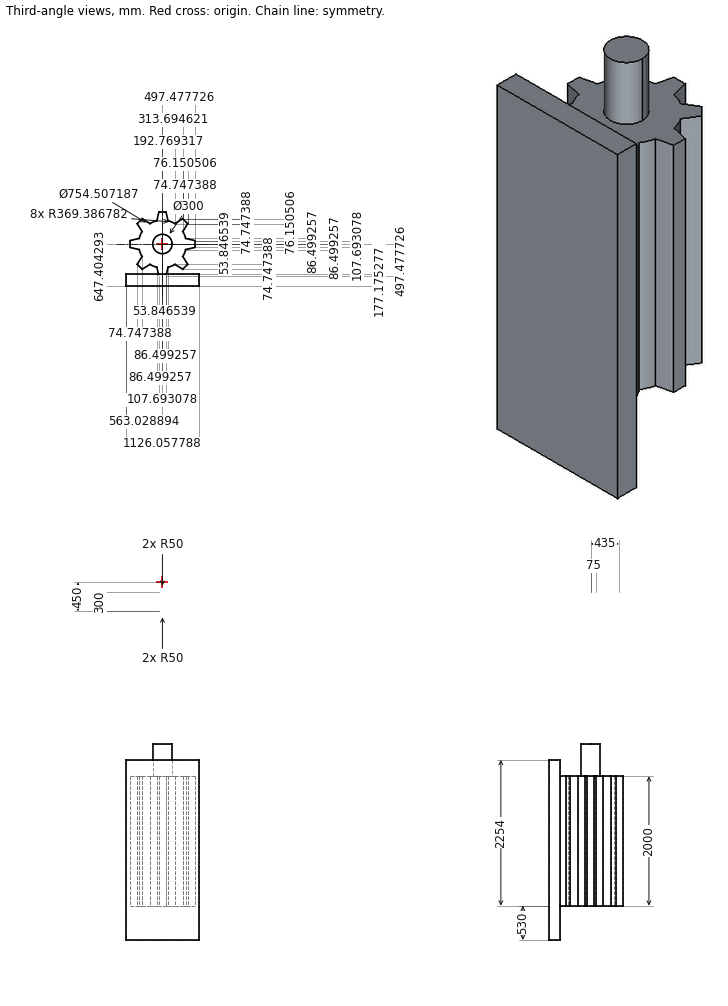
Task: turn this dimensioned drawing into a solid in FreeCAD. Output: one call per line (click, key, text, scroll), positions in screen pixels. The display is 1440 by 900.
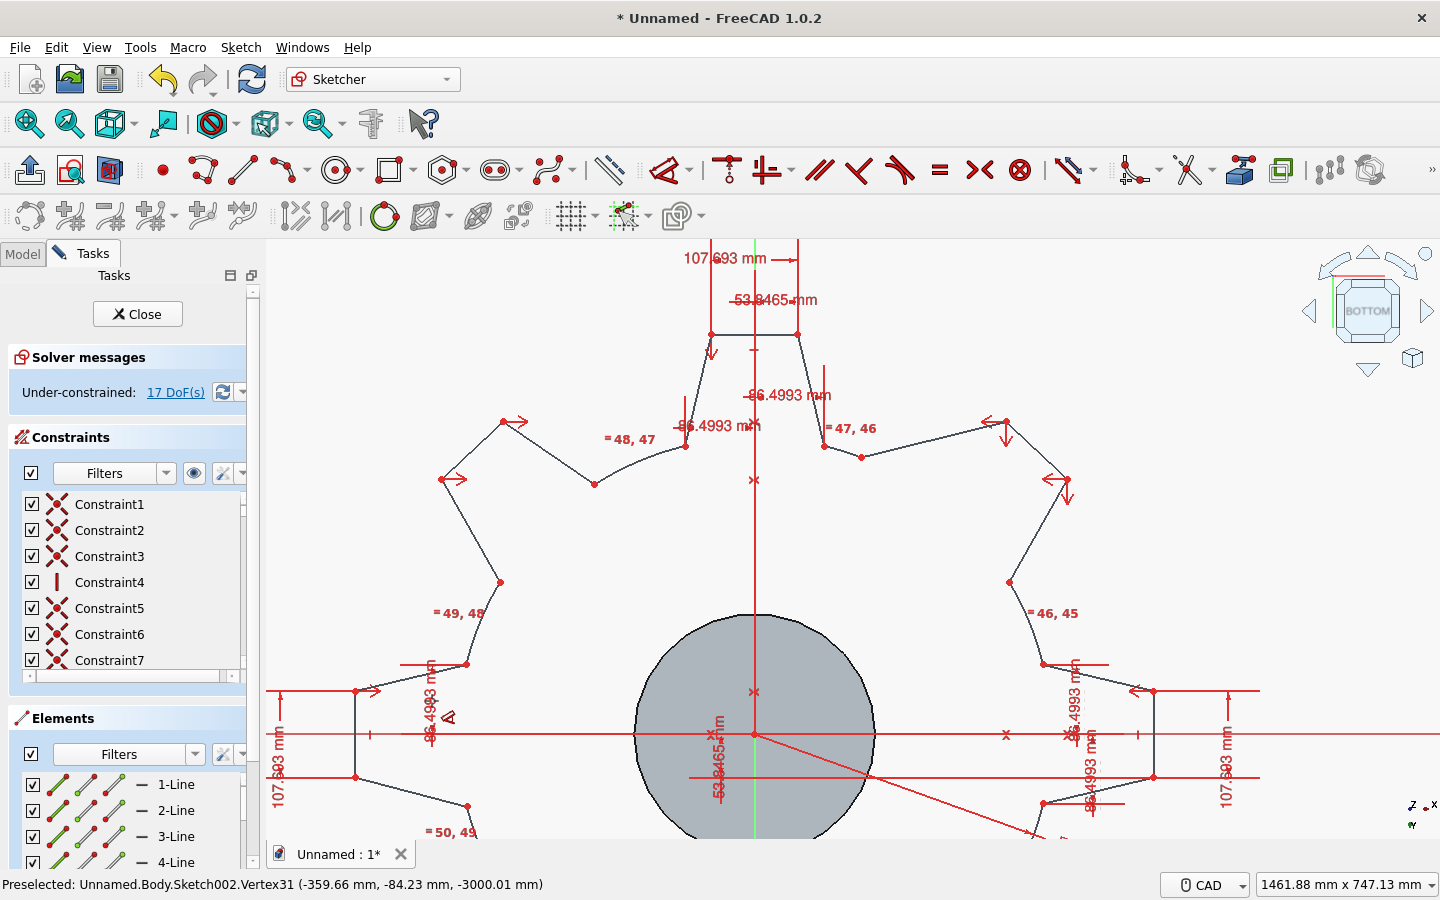
click(467, 807)
click(433, 771)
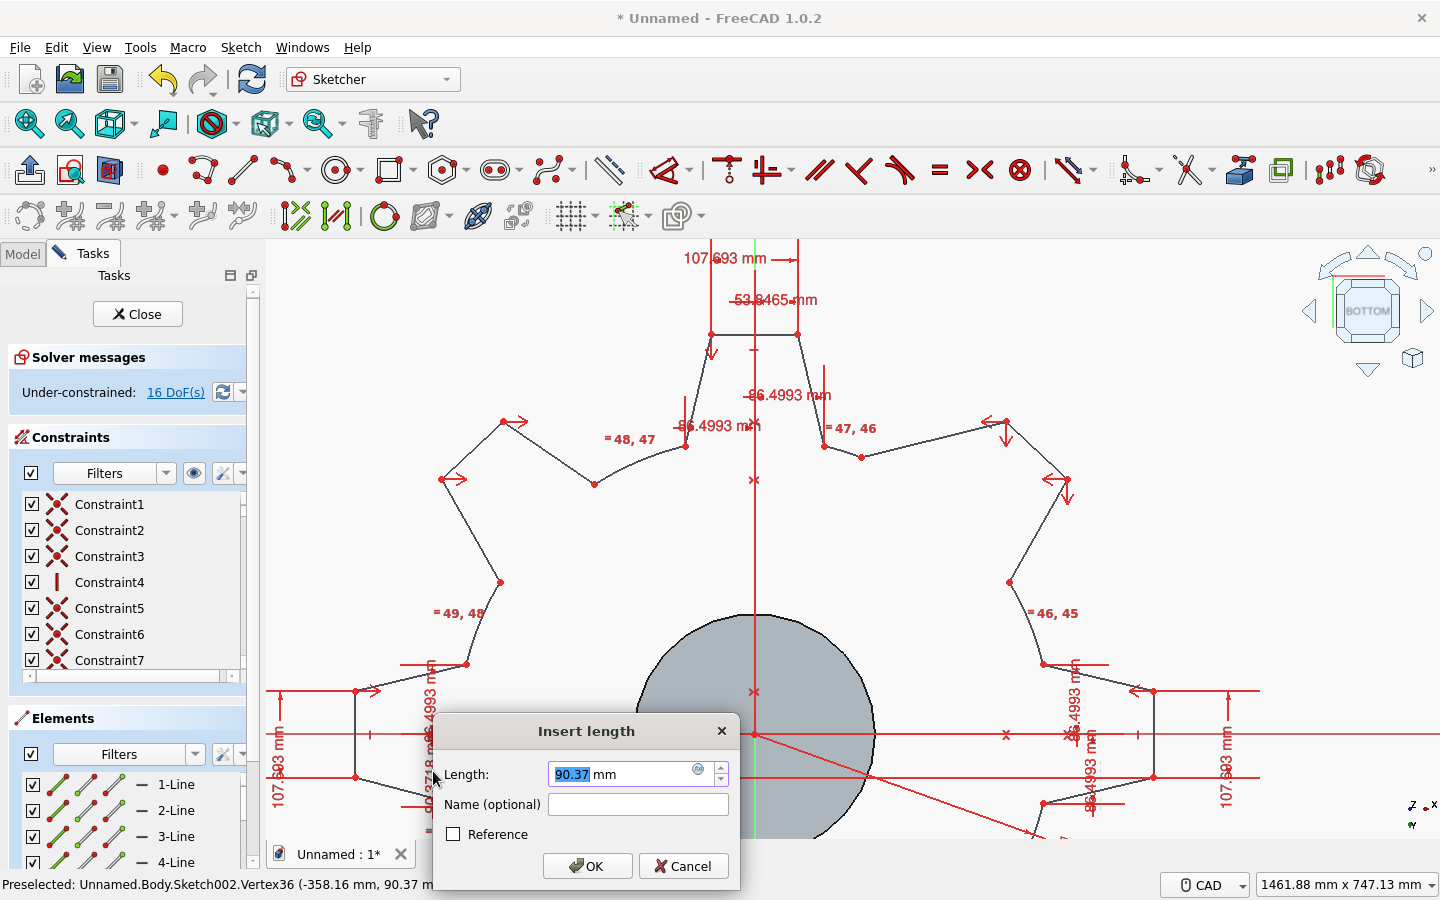
text(86.499257)
key(Return)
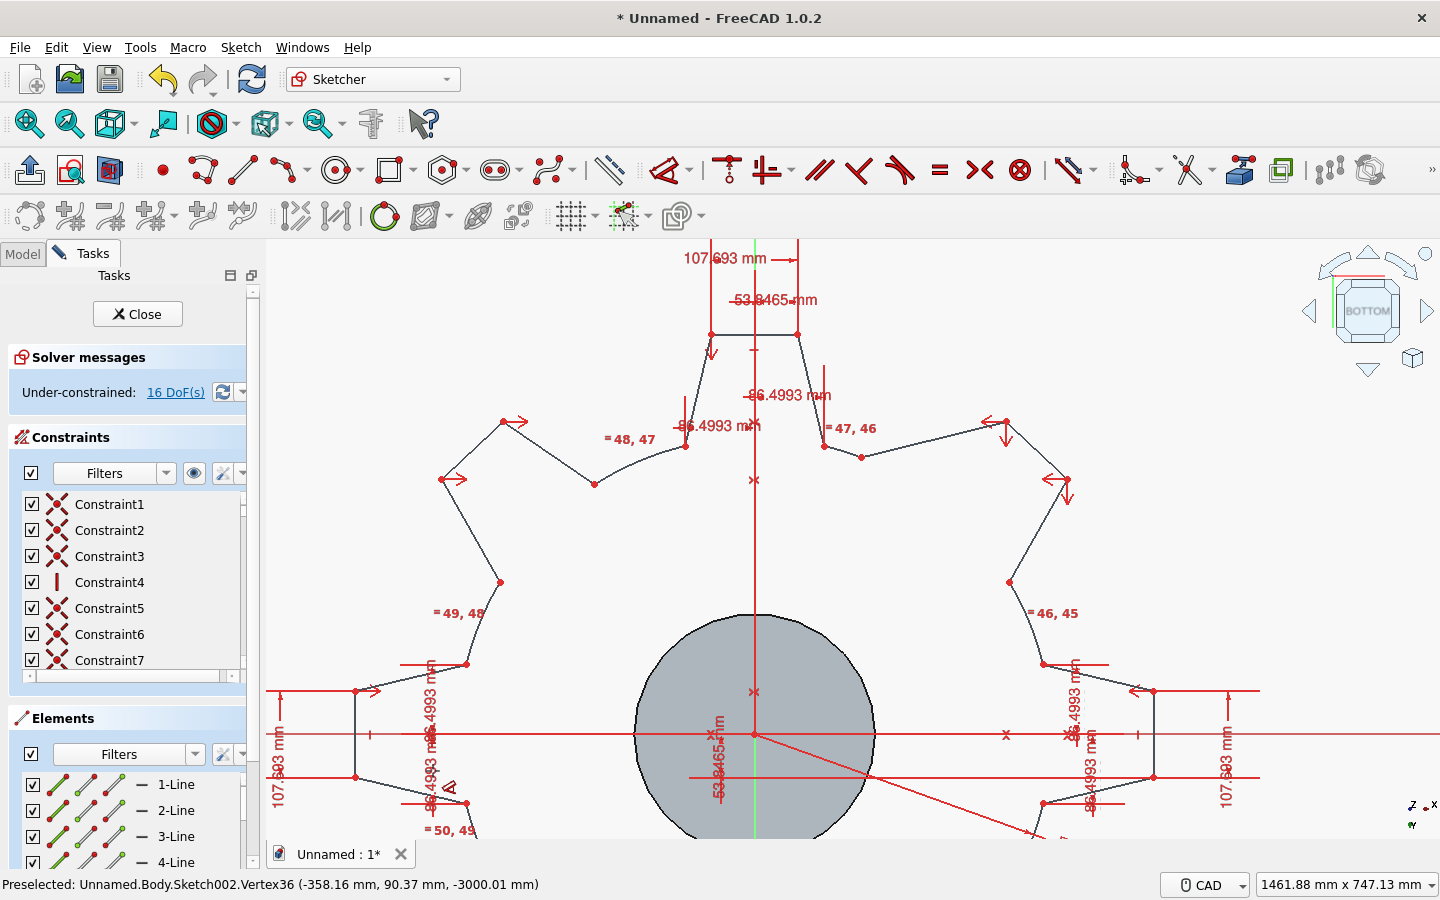
scroll(809, 380, down, 4)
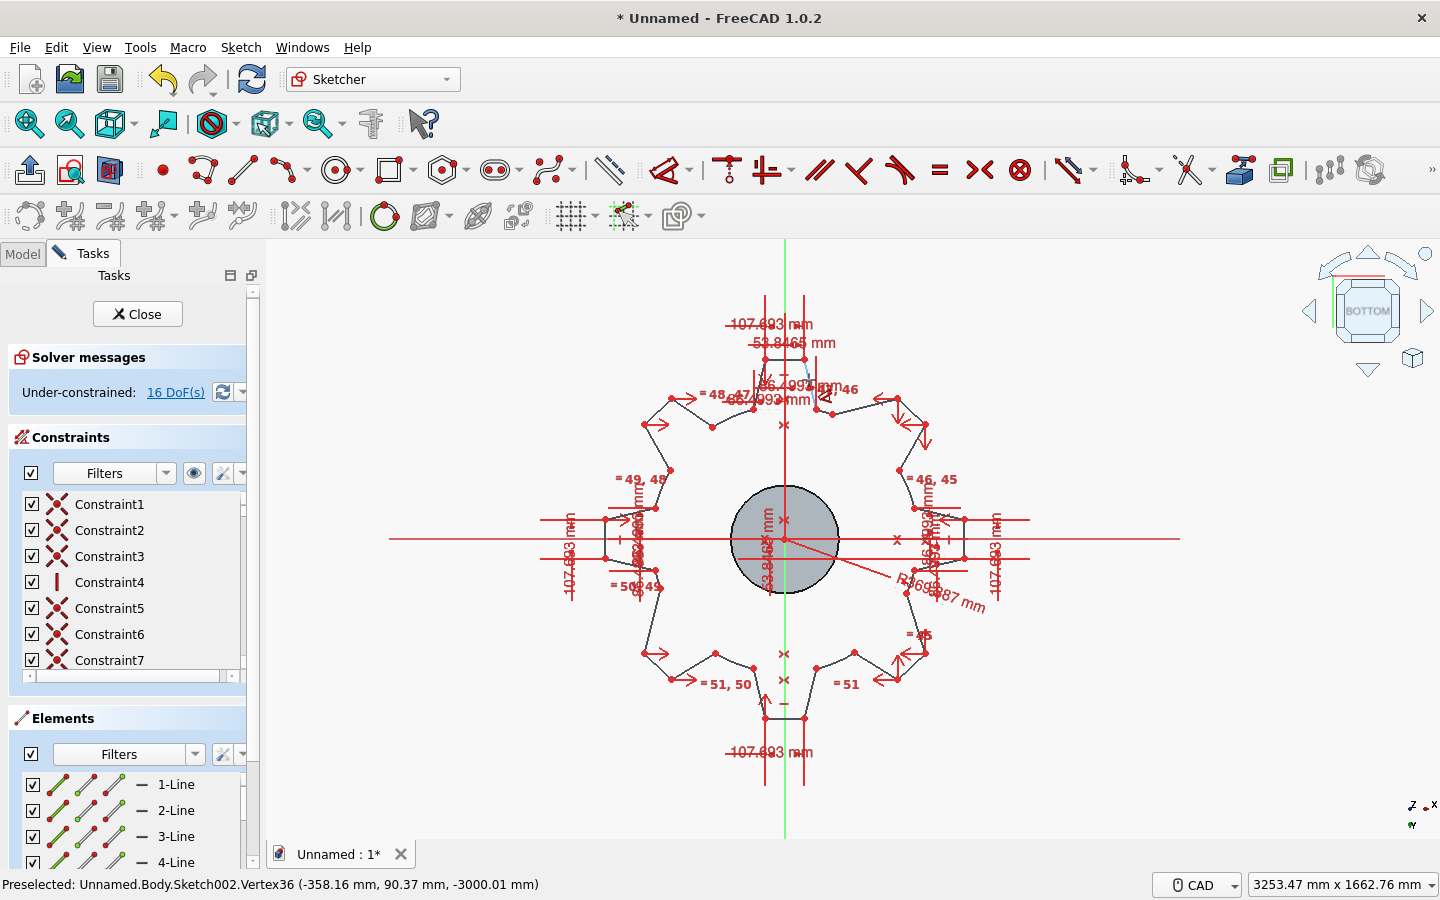
scroll(754, 669, up, 2)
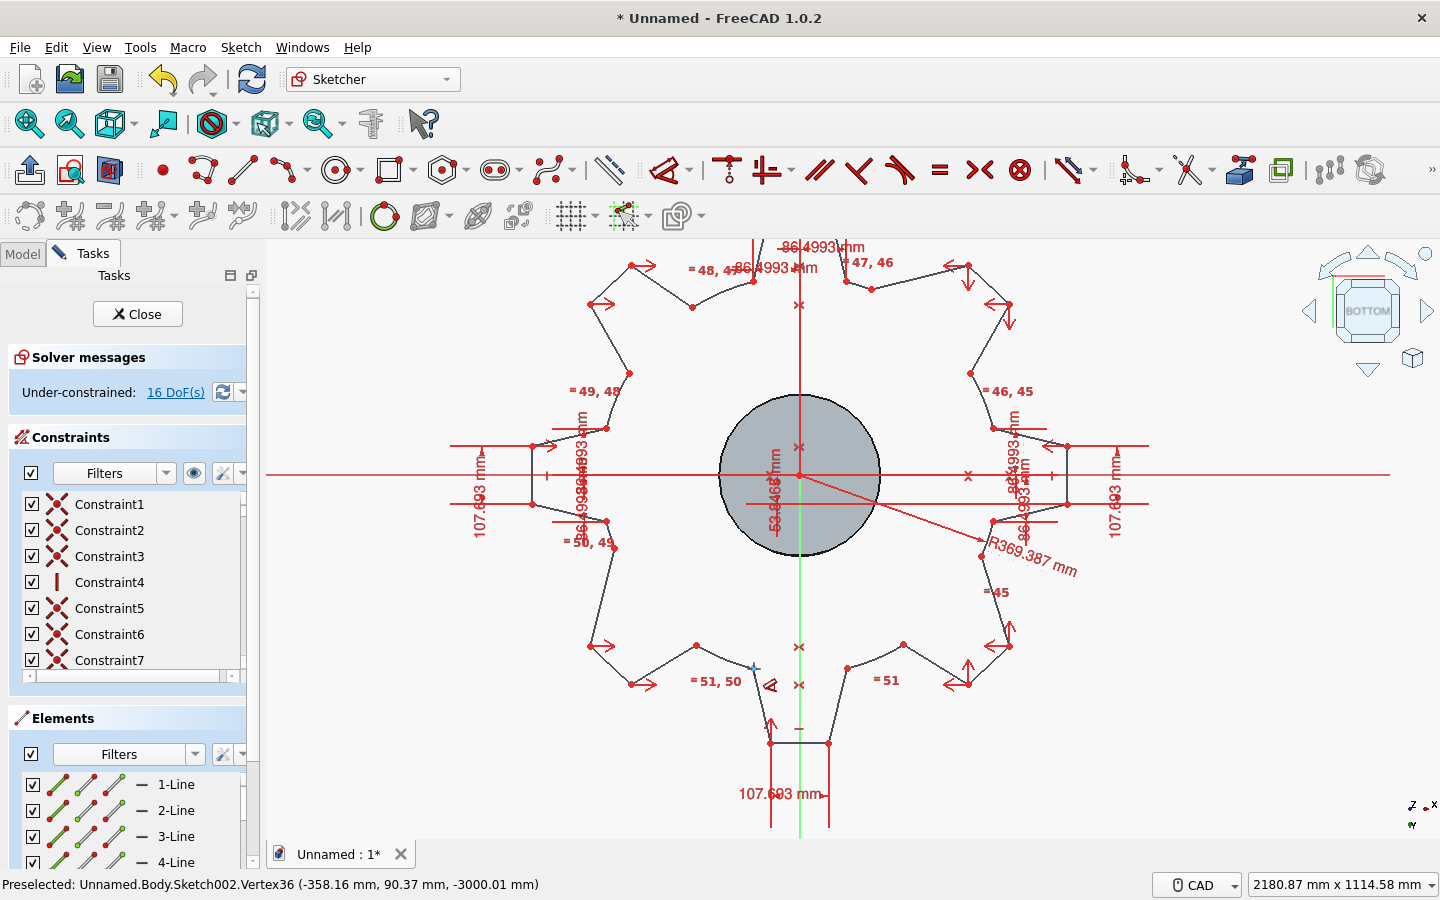
click(753, 669)
click(776, 703)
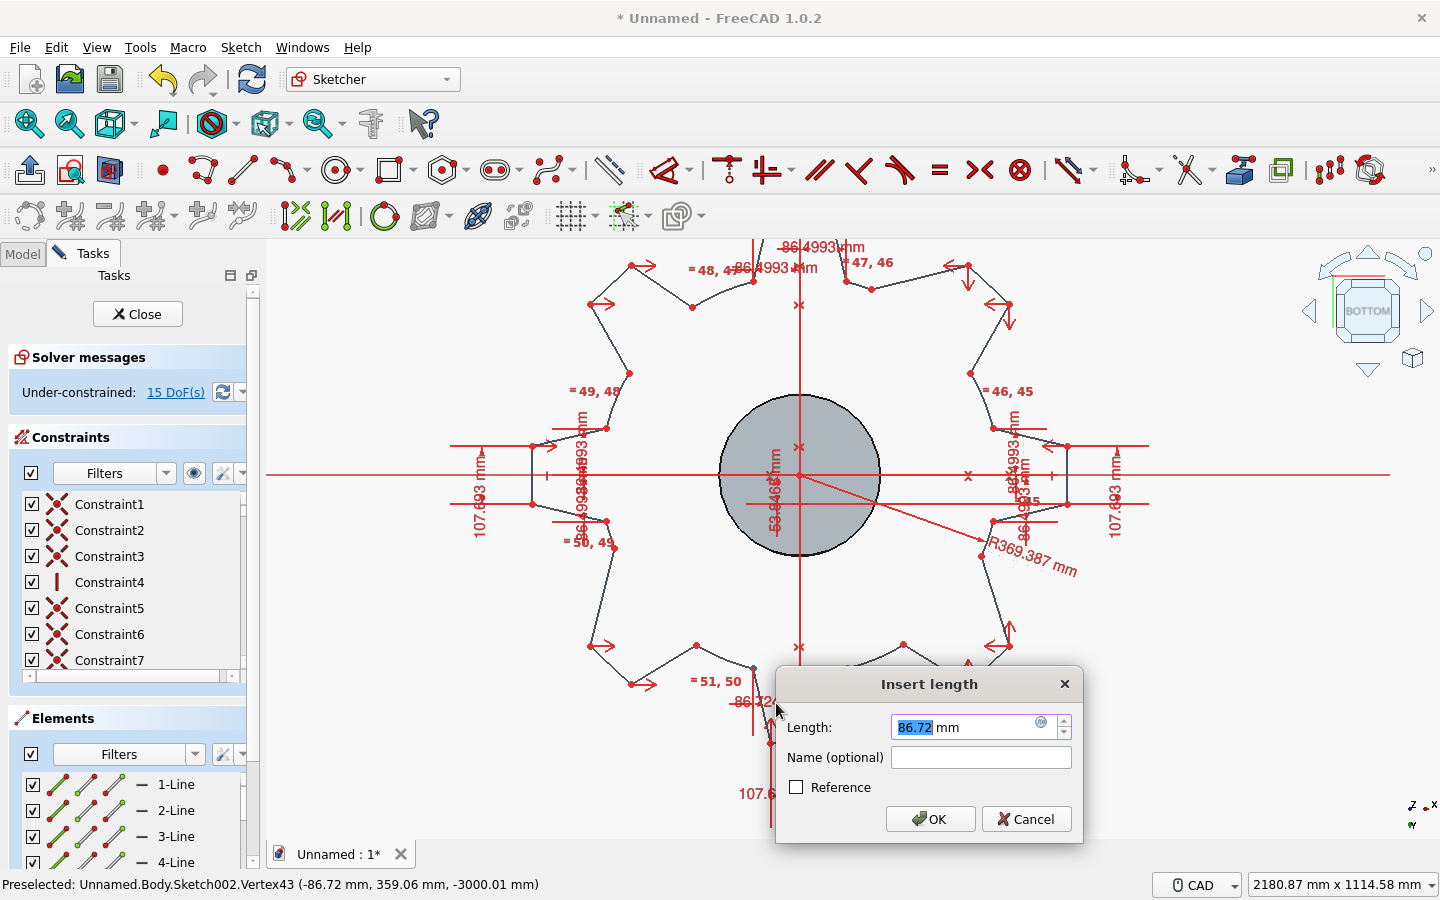
text(86.499257)
key(Return)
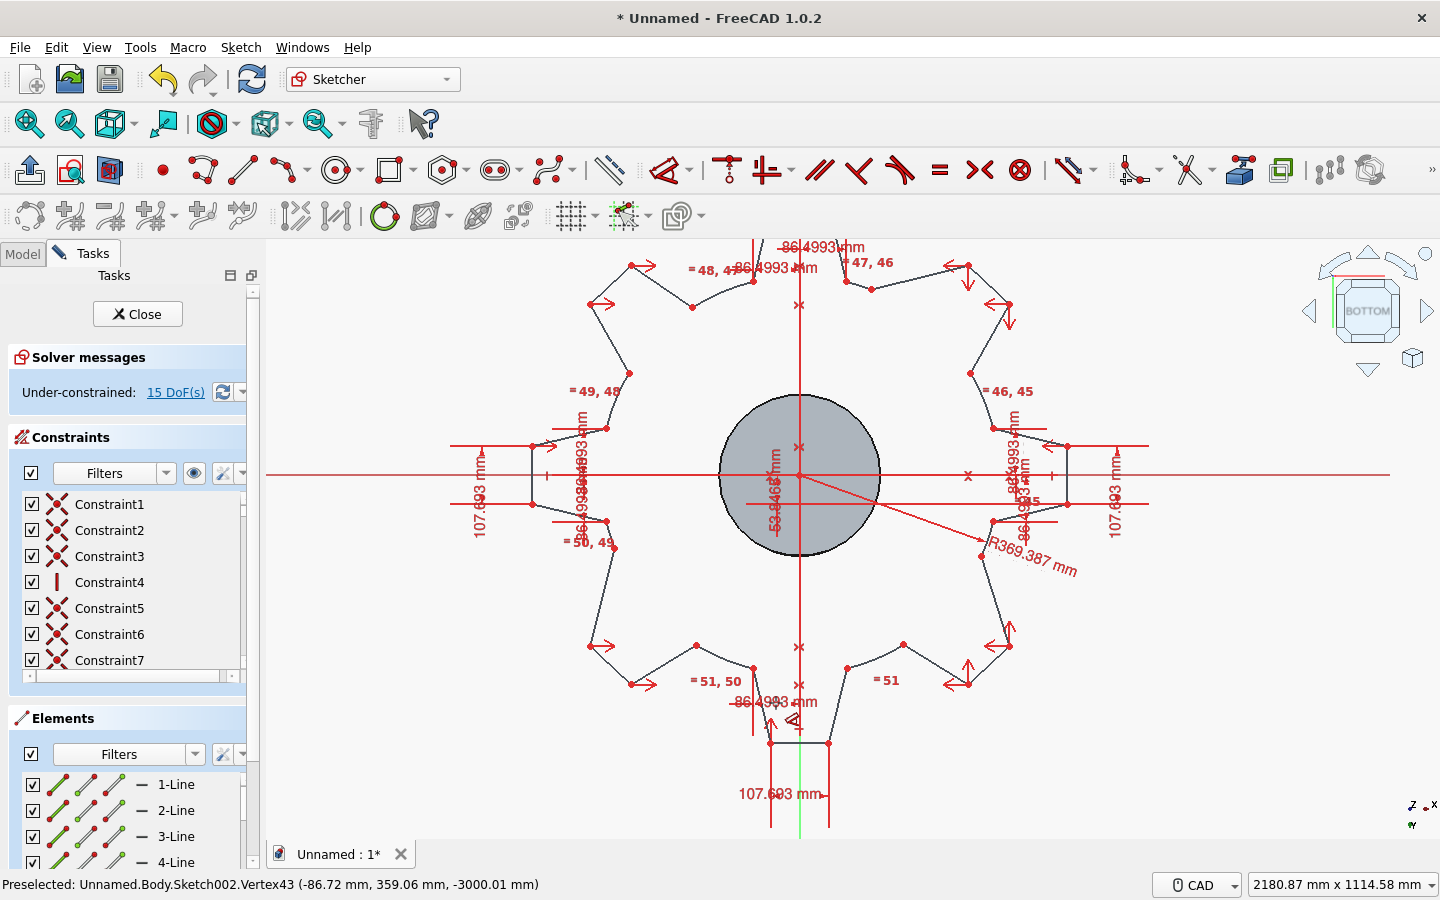
click(847, 668)
click(823, 441)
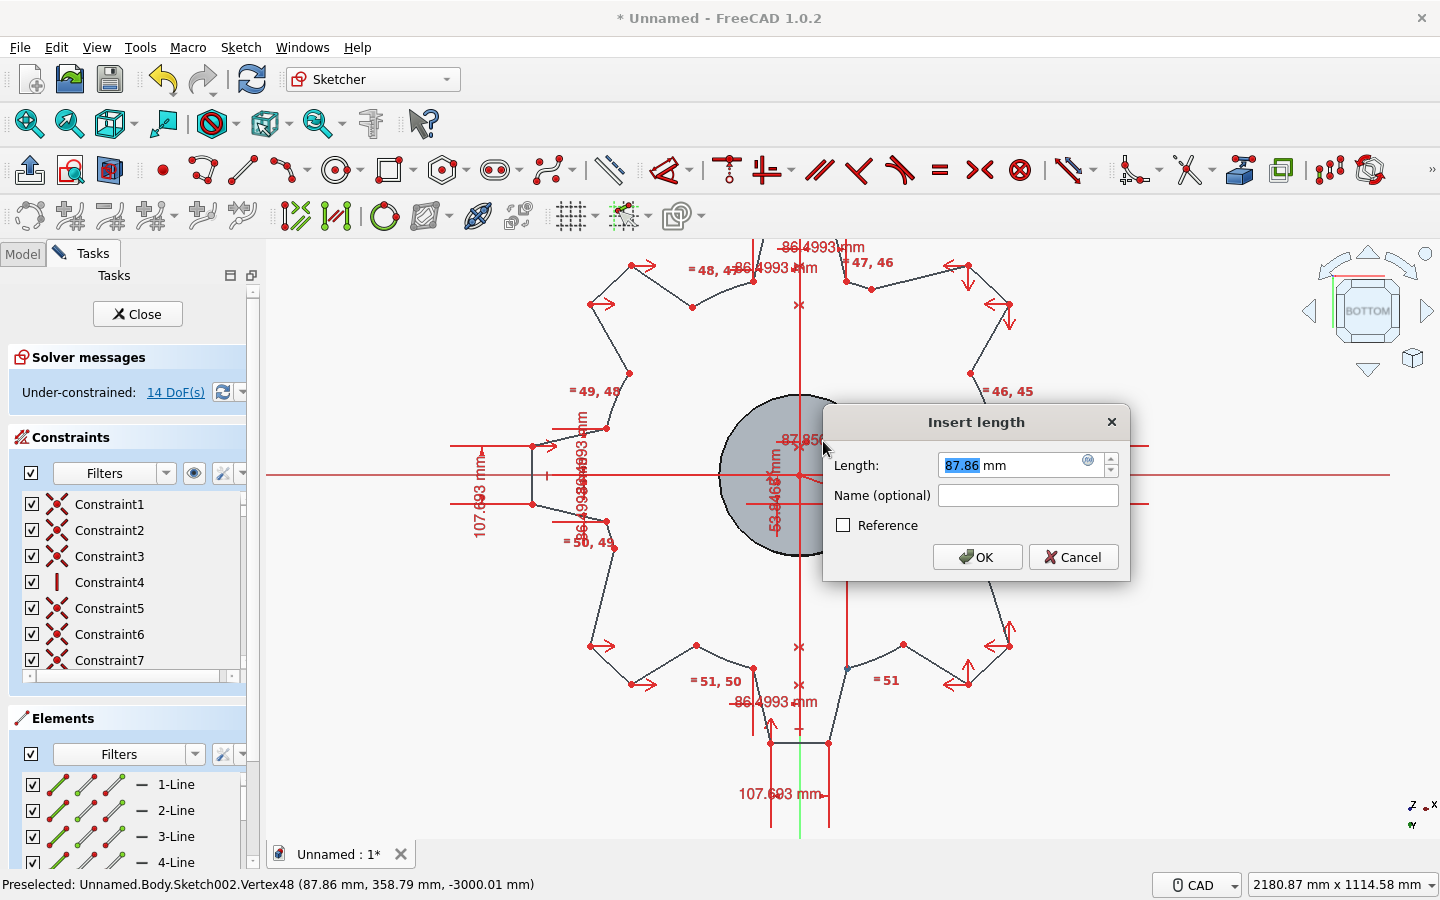
text(86.499257)
key(Return)